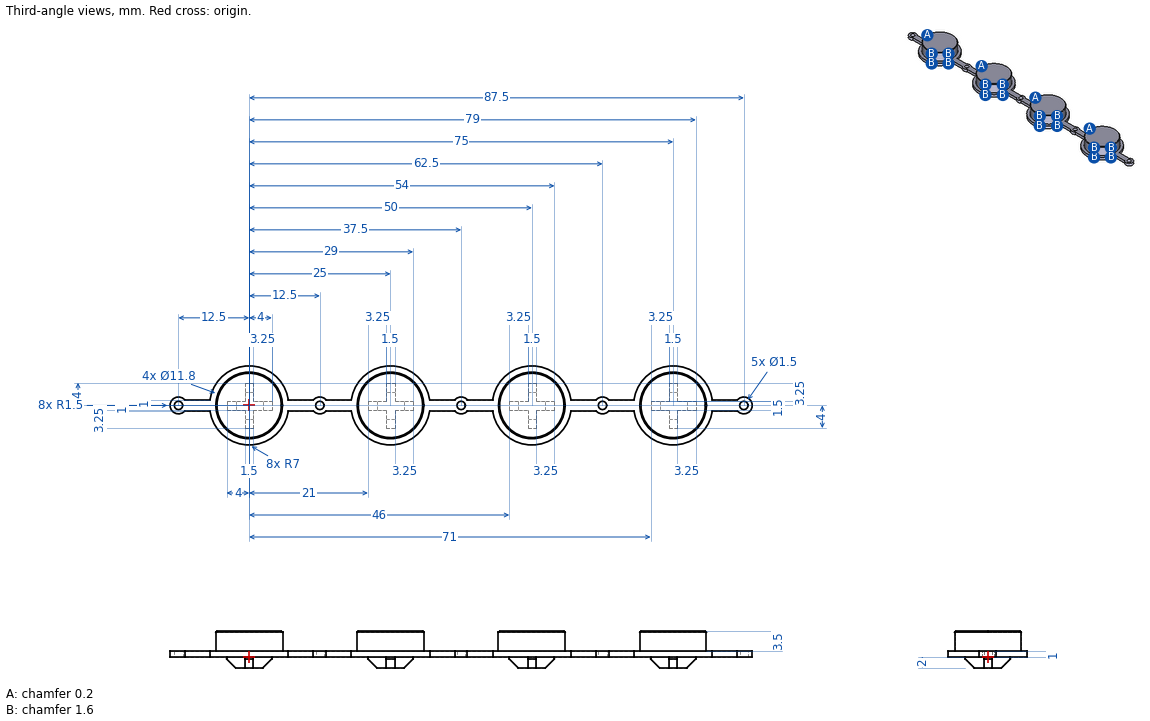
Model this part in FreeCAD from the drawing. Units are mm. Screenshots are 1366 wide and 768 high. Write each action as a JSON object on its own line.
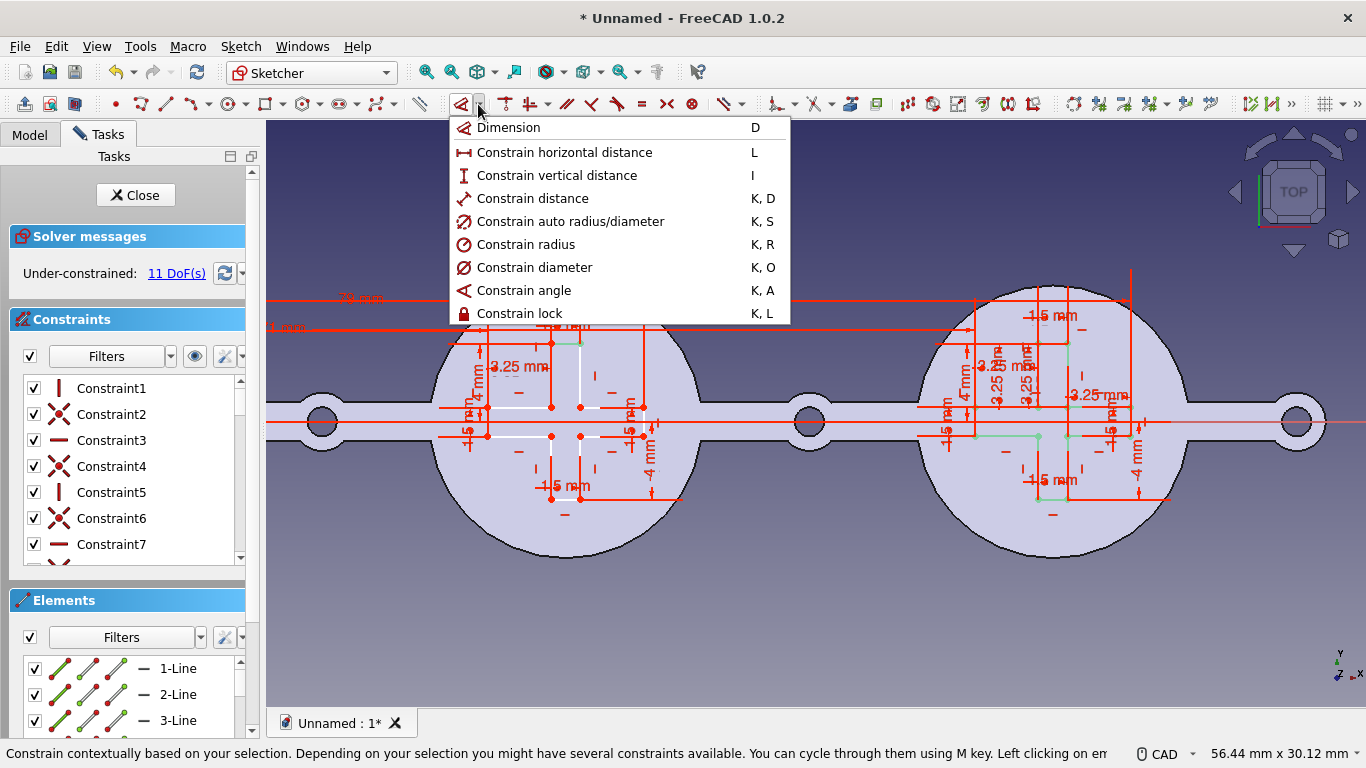
{"action": "left_click", "coordinate": [620, 176]}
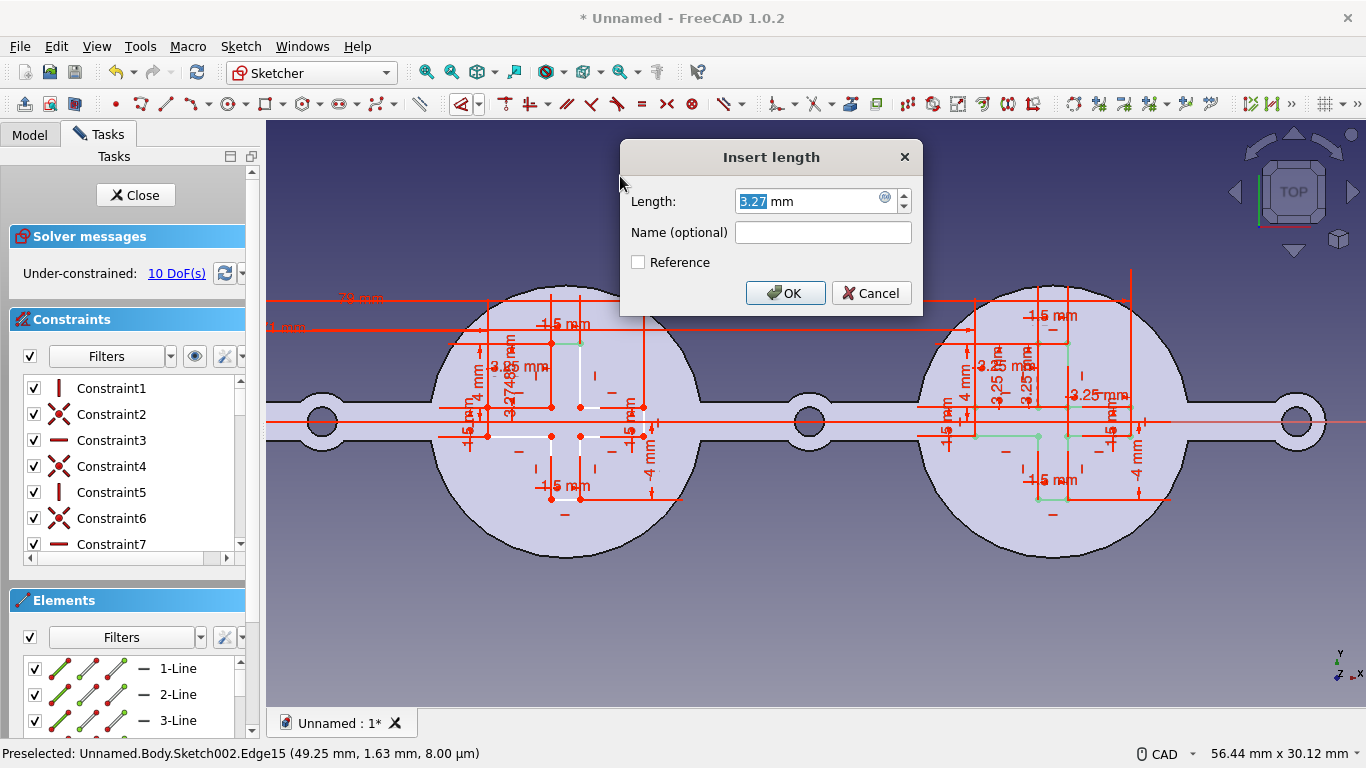
{"action": "type", "text": "3.25"}
{"action": "key", "text": "Return"}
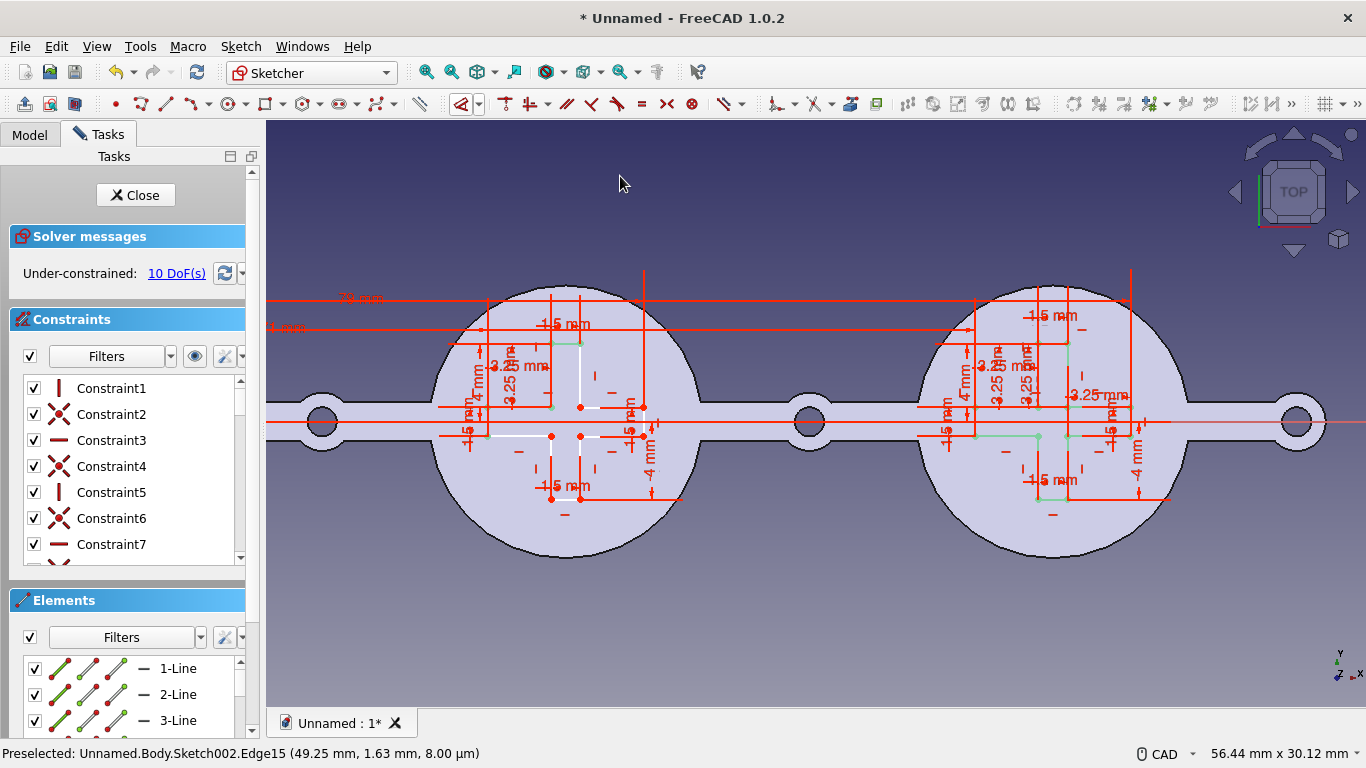
{"action": "left_click", "coordinate": [580, 363]}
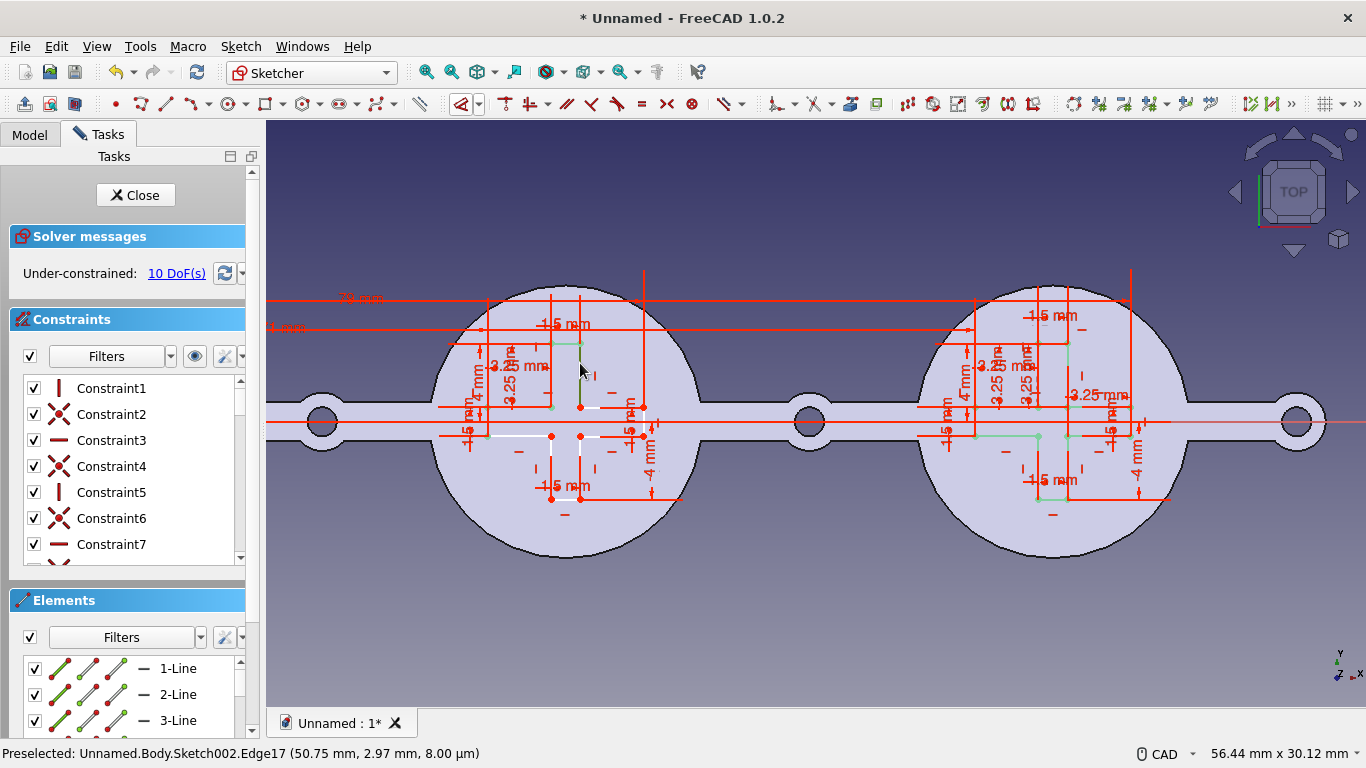
{"action": "left_click", "coordinate": [478, 104]}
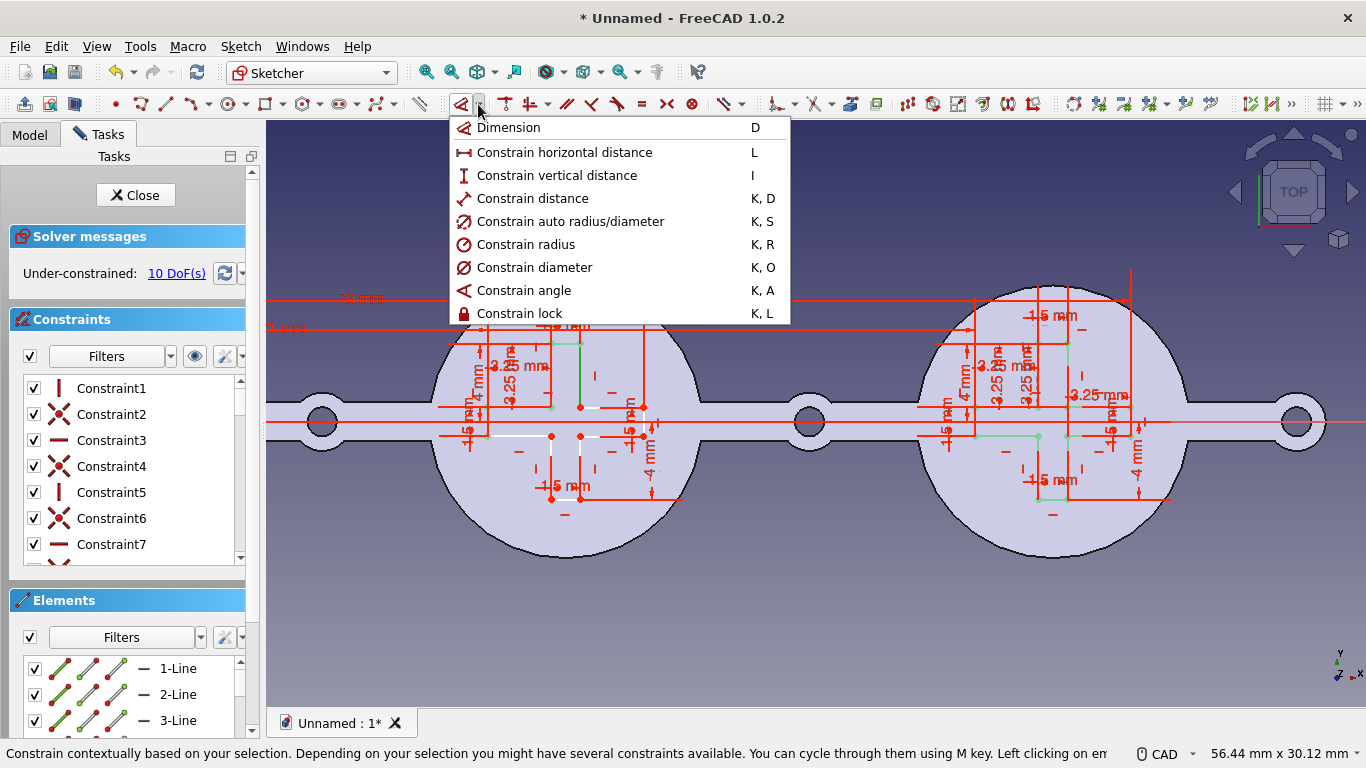
{"action": "left_click", "coordinate": [620, 176]}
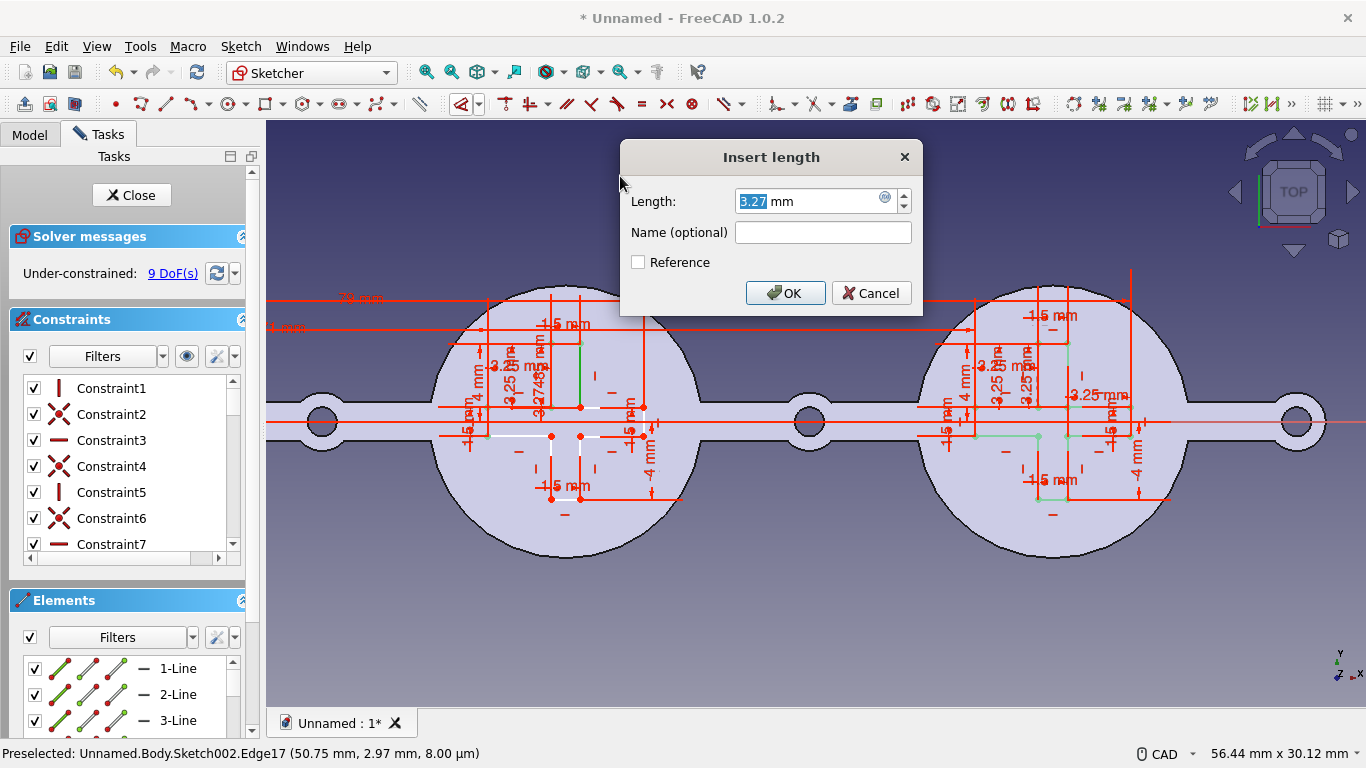
{"action": "type", "text": "3.25"}
{"action": "key", "text": "Return"}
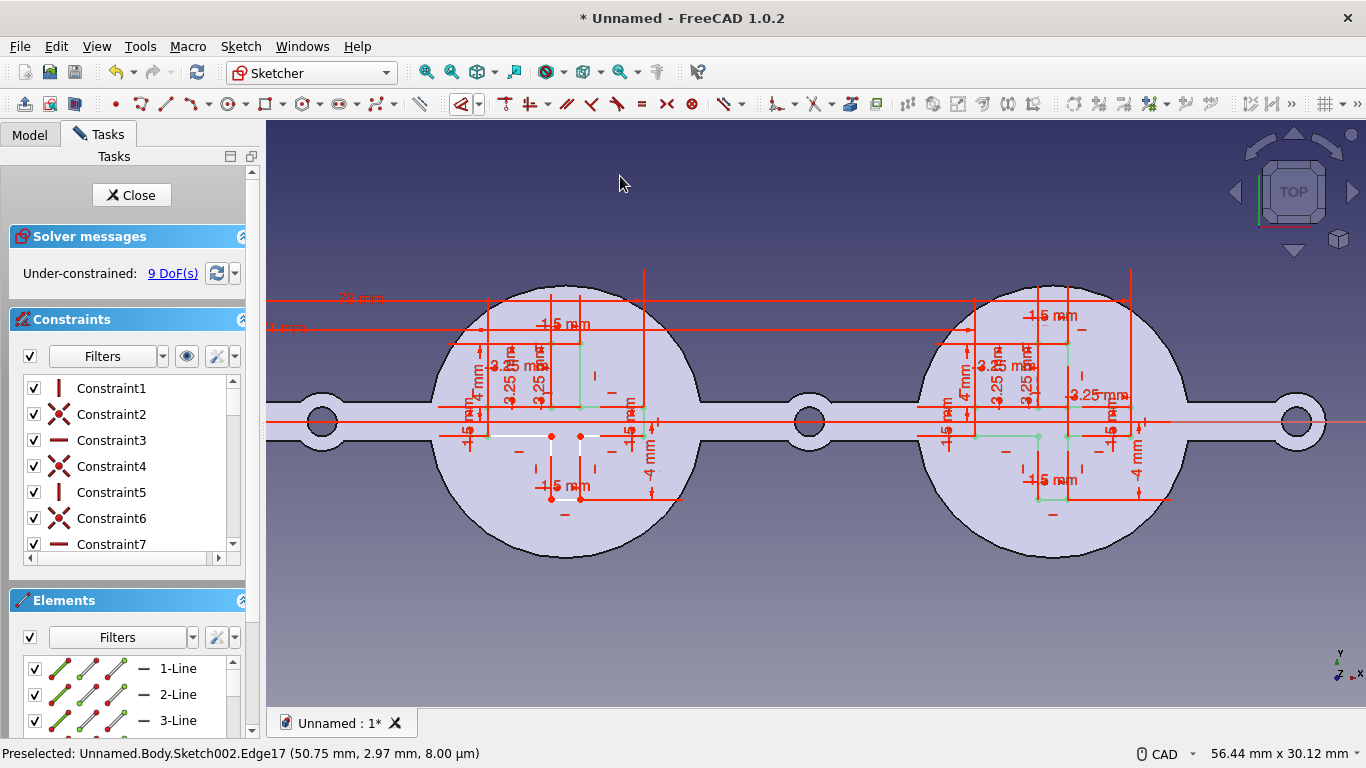
{"action": "left_click", "coordinate": [599, 436]}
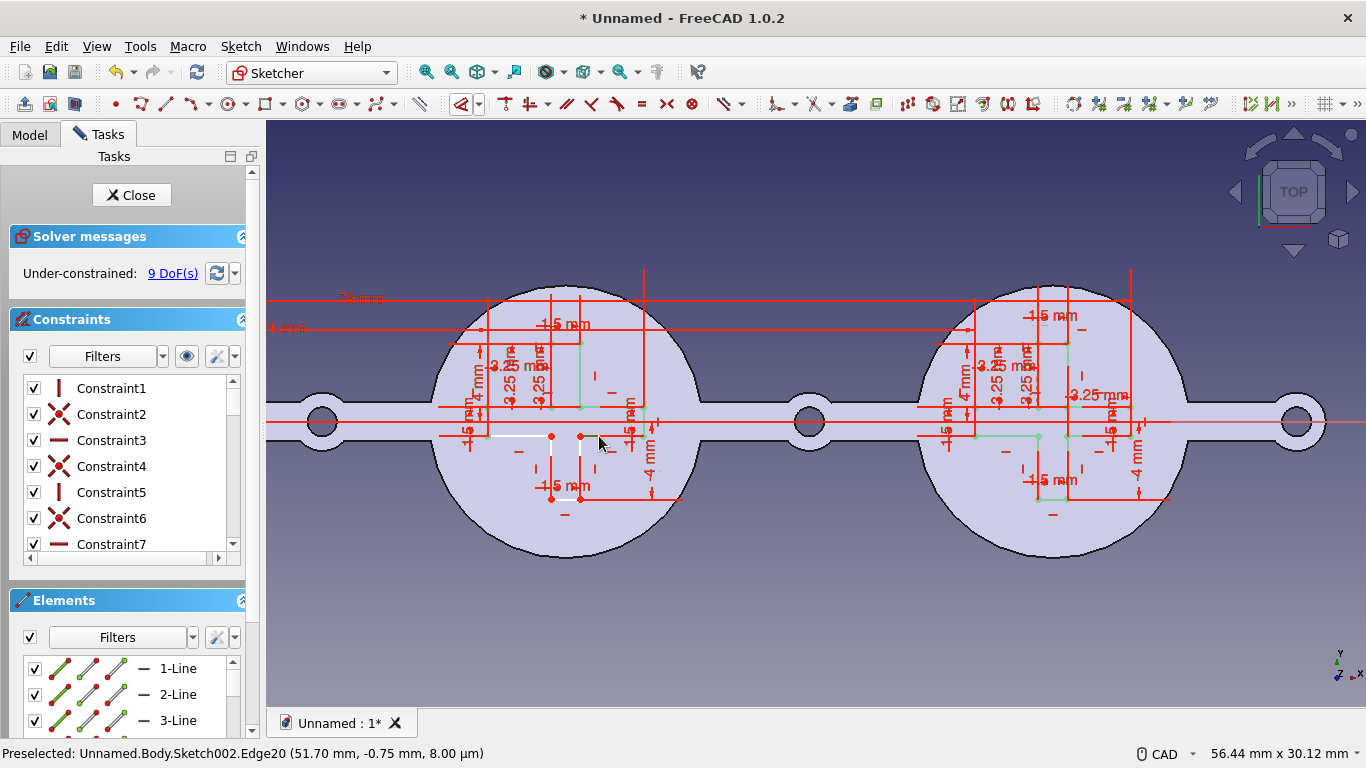
{"action": "key", "text": "l"}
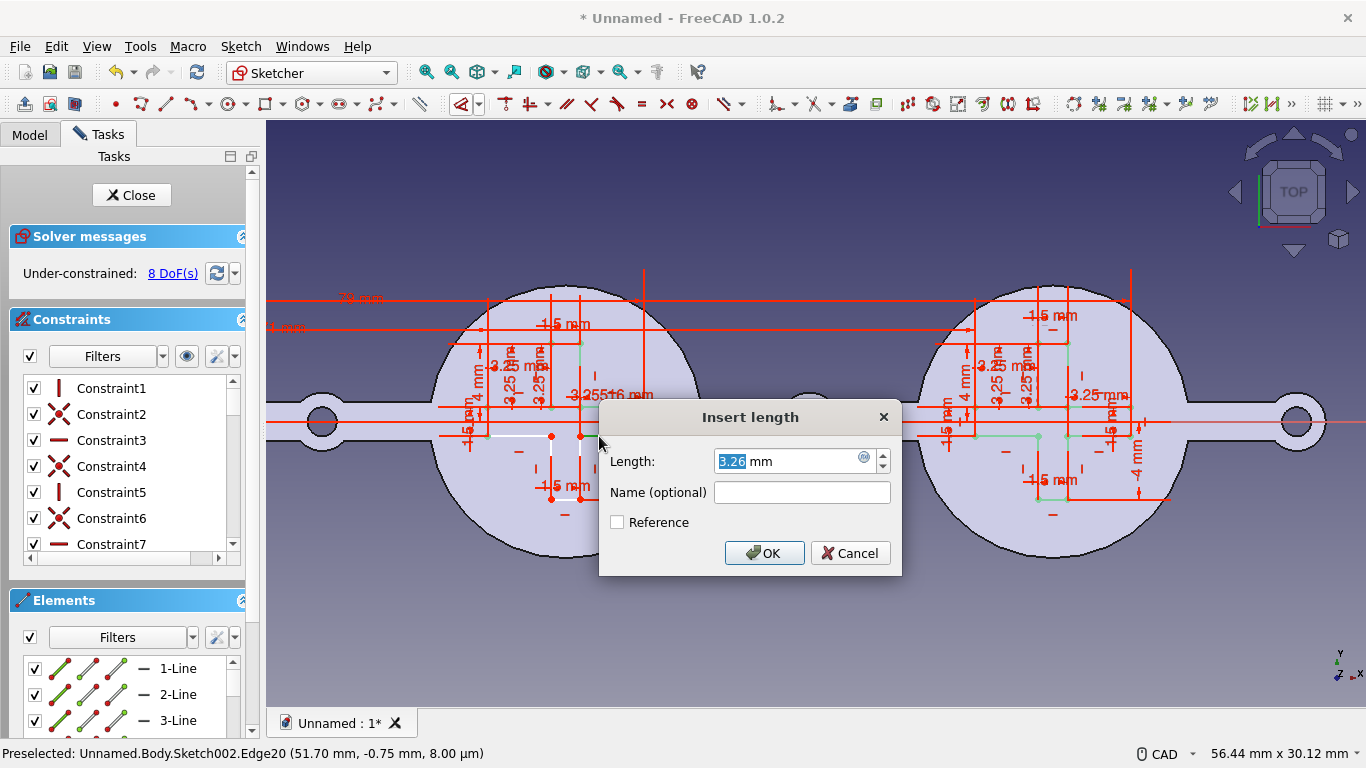
{"action": "type", "text": "3.25"}
{"action": "key", "text": "Return"}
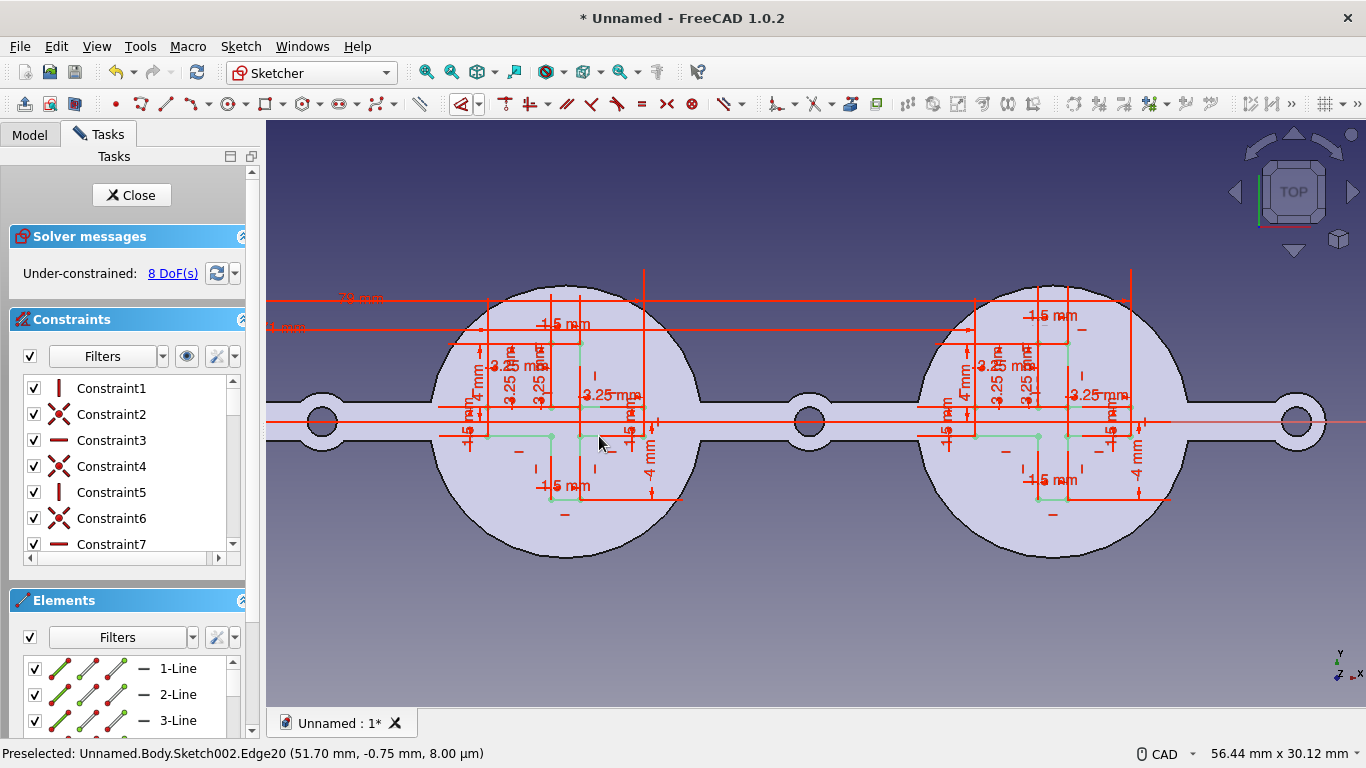
{"action": "scroll", "coordinate": [995, 409], "scroll_direction": "down", "scroll_amount": 5}